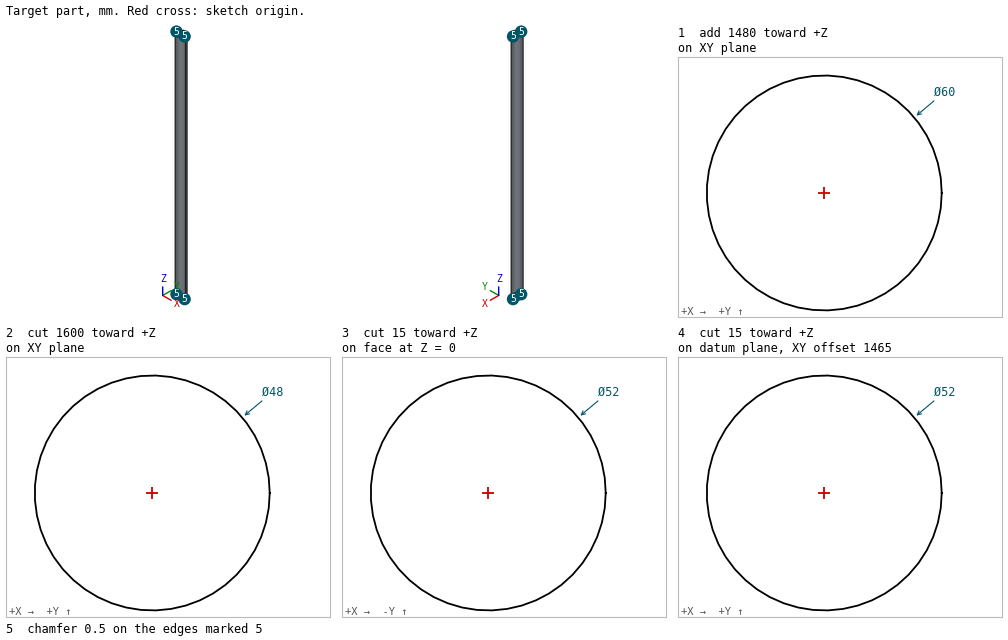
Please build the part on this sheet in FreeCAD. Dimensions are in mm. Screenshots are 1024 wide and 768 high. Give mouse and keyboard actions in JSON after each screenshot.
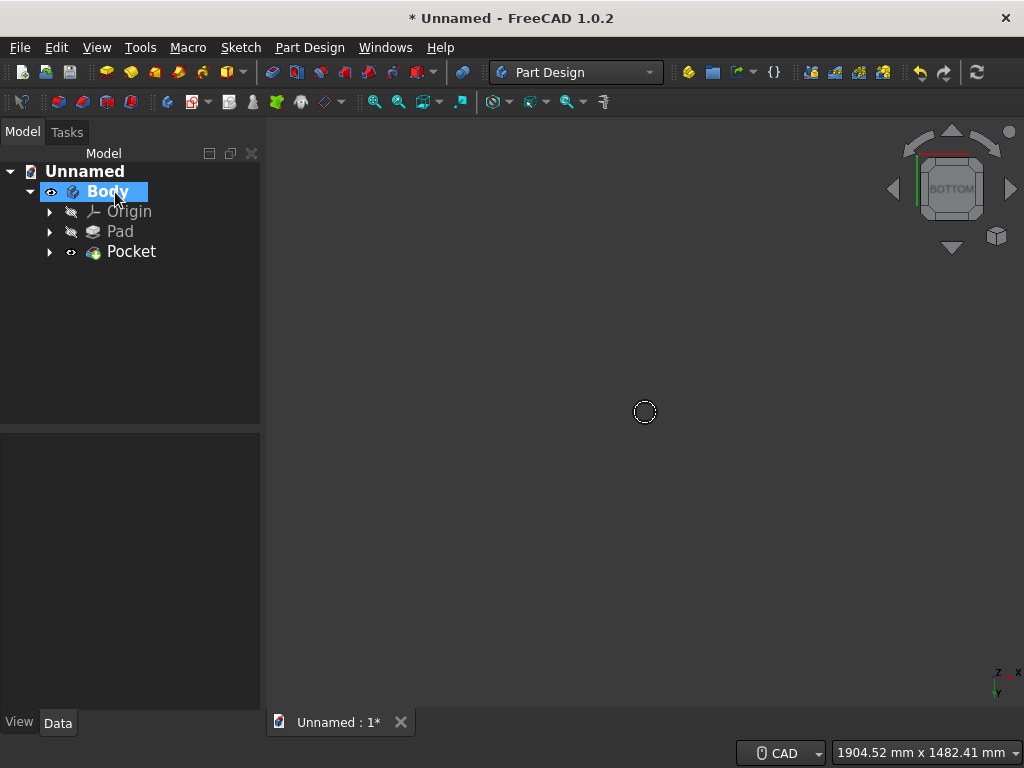
{"action": "left_click", "coordinate": [376, 102]}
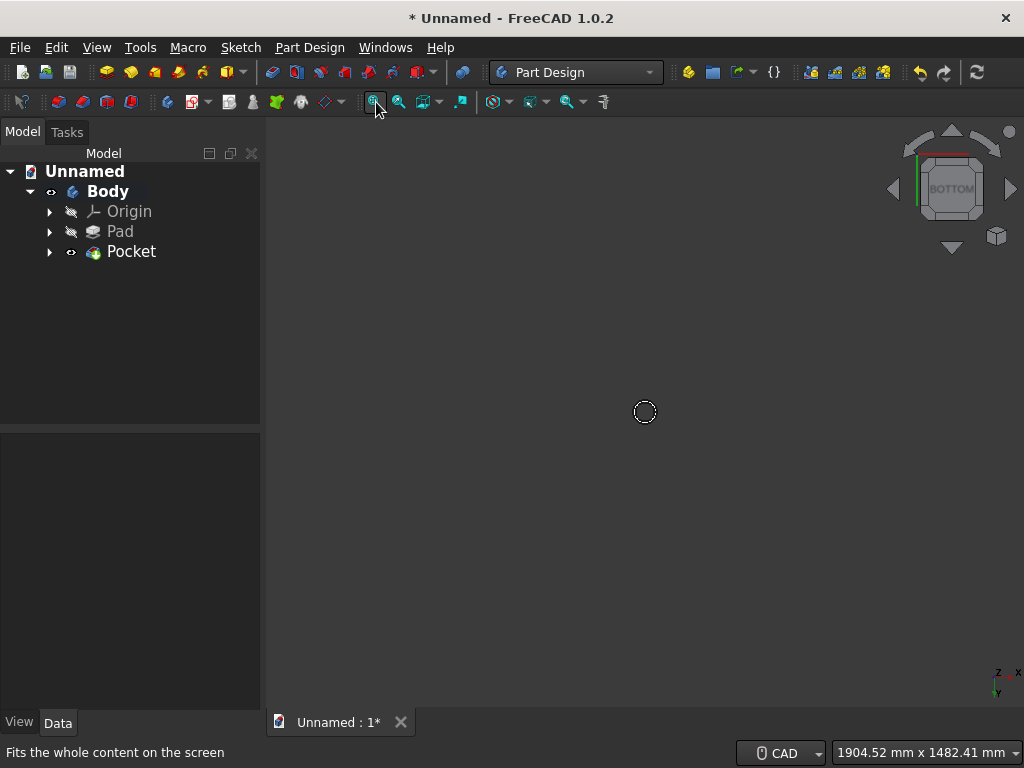
{"action": "scroll", "coordinate": [648, 421], "scroll_direction": "up", "scroll_amount": 12}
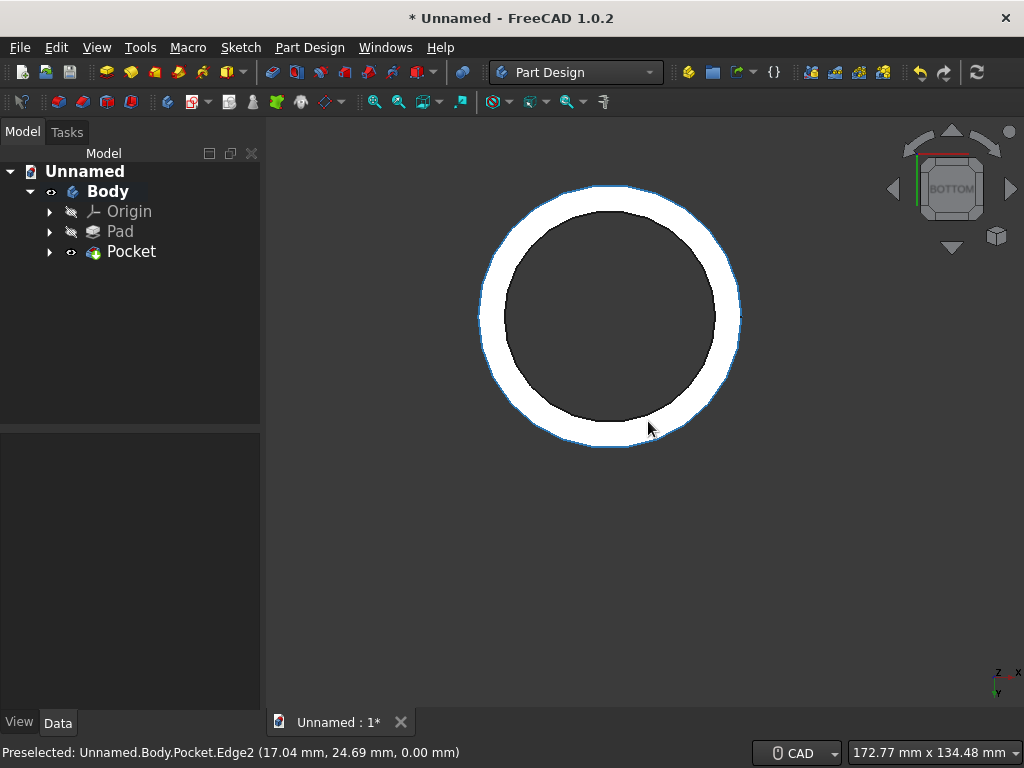
{"action": "left_click", "coordinate": [647, 428]}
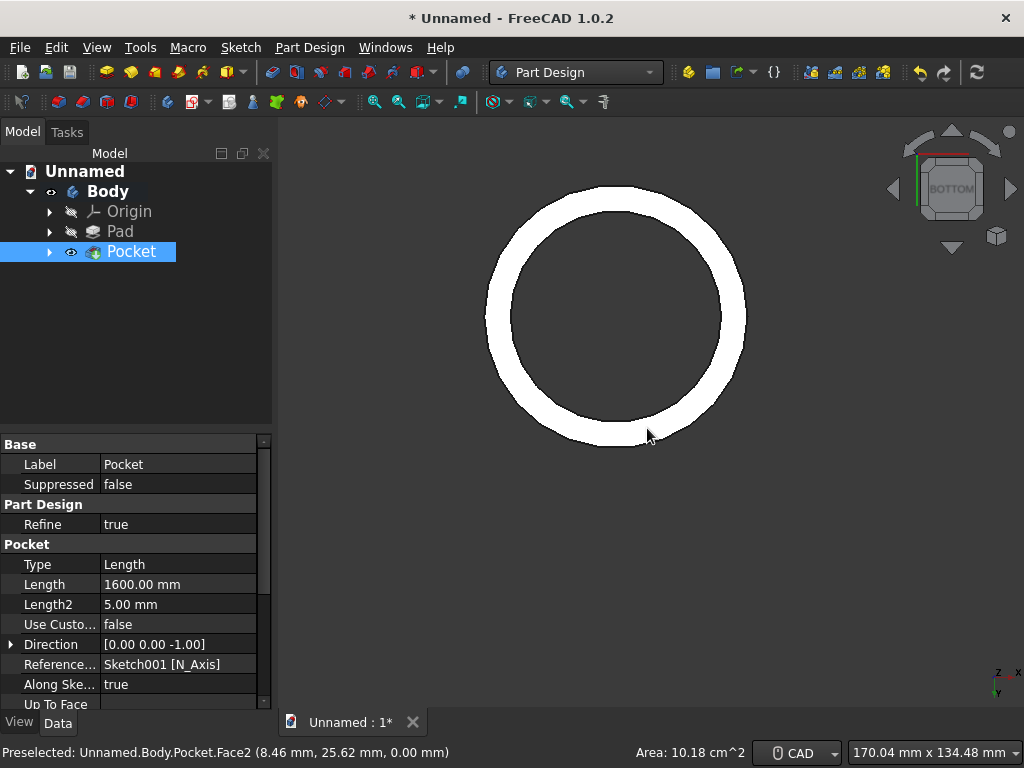
{"action": "left_click", "coordinate": [192, 102]}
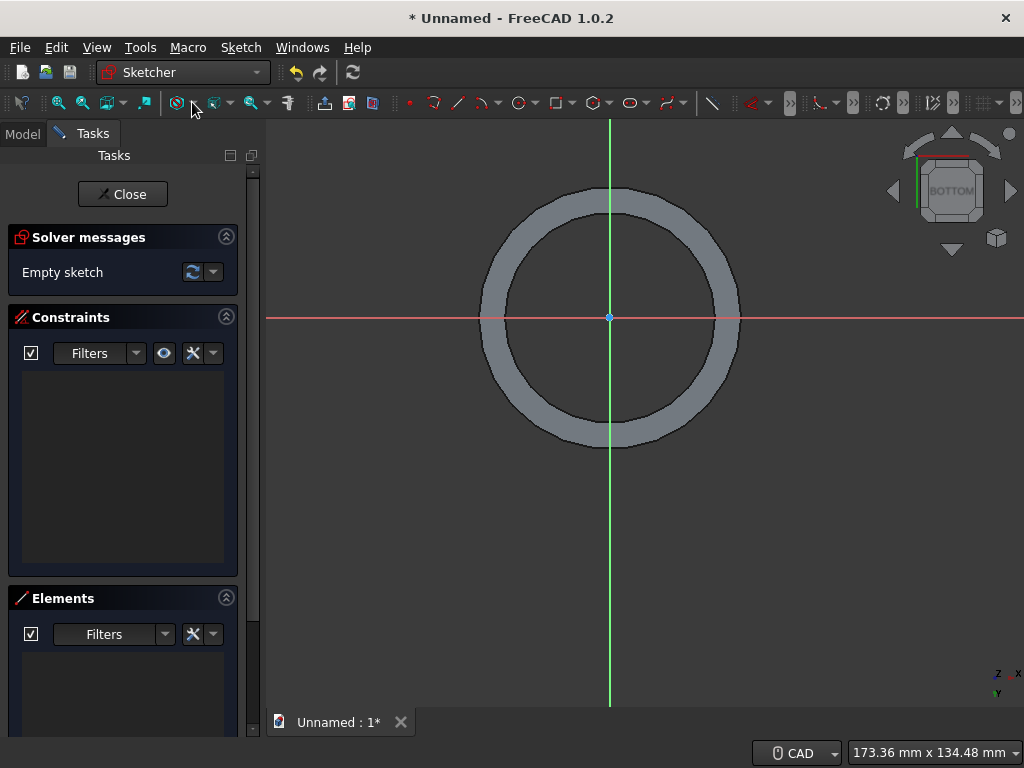
{"action": "scroll", "coordinate": [651, 202], "scroll_direction": "up", "scroll_amount": 3}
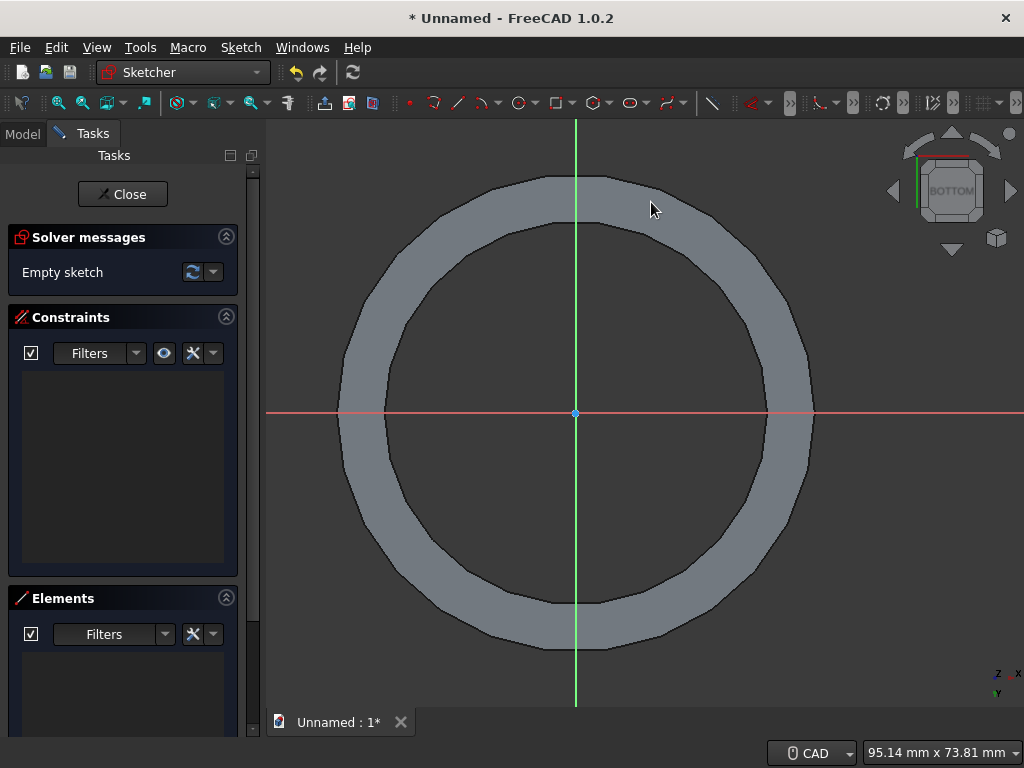
{"action": "left_click", "coordinate": [520, 104]}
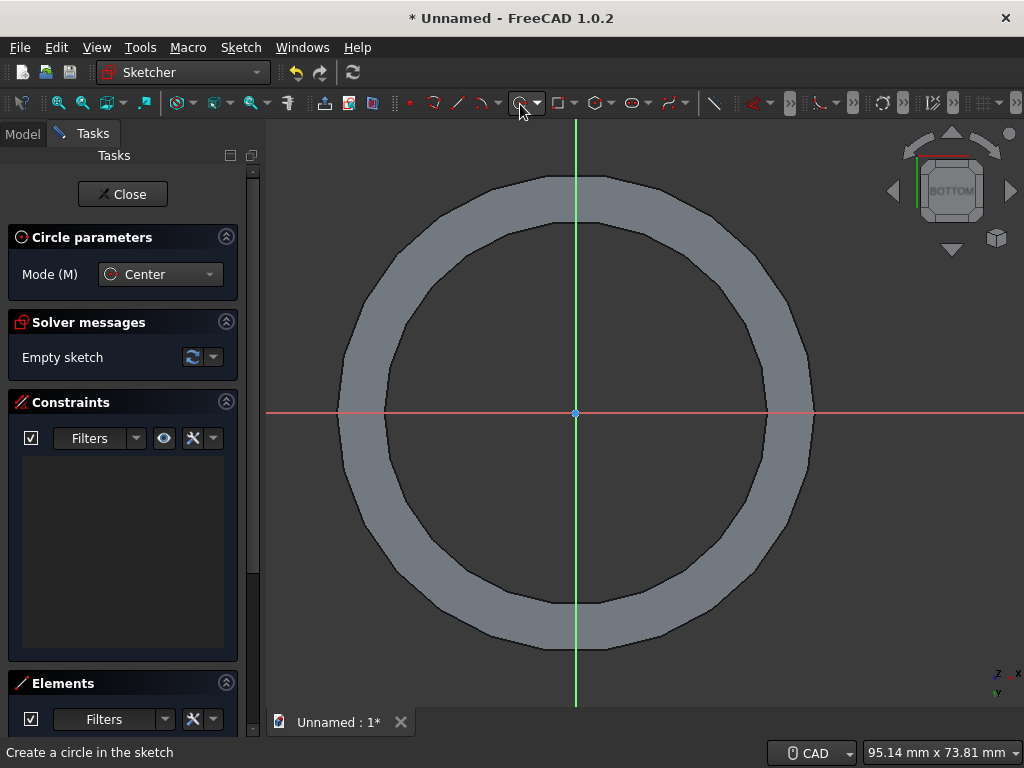
{"action": "left_click", "coordinate": [576, 413]}
{"action": "mouse_move", "coordinate": [722, 267]}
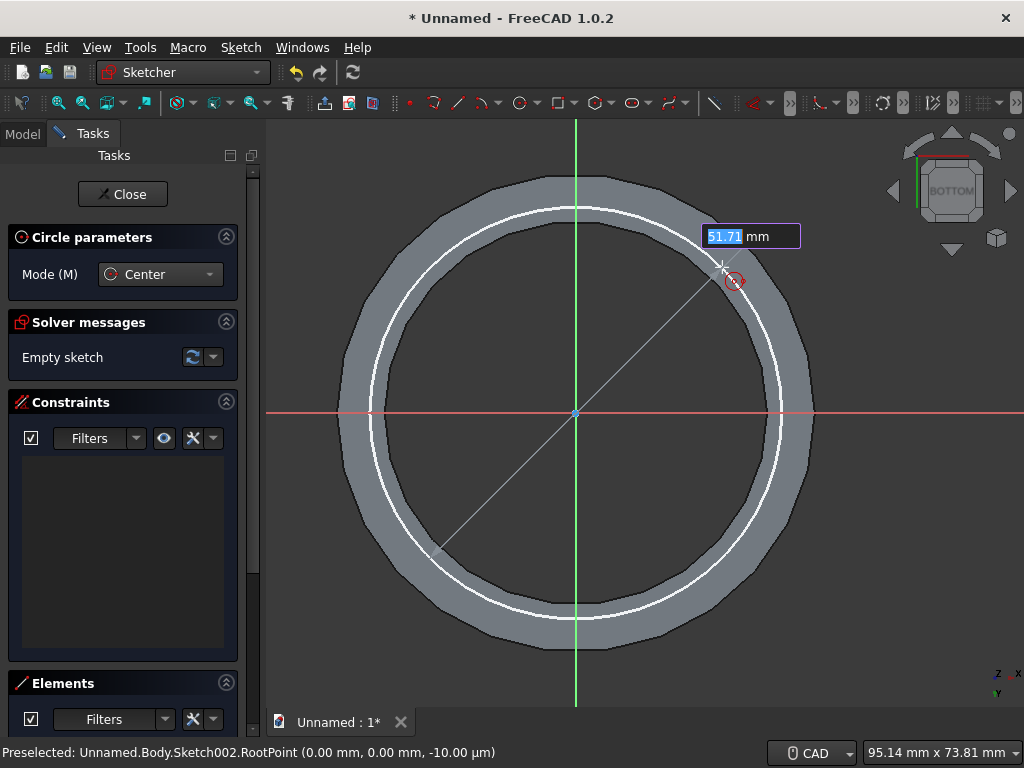
{"action": "type", "text": "52"}
{"action": "key", "text": "Return"}
{"action": "key", "text": "Escape"}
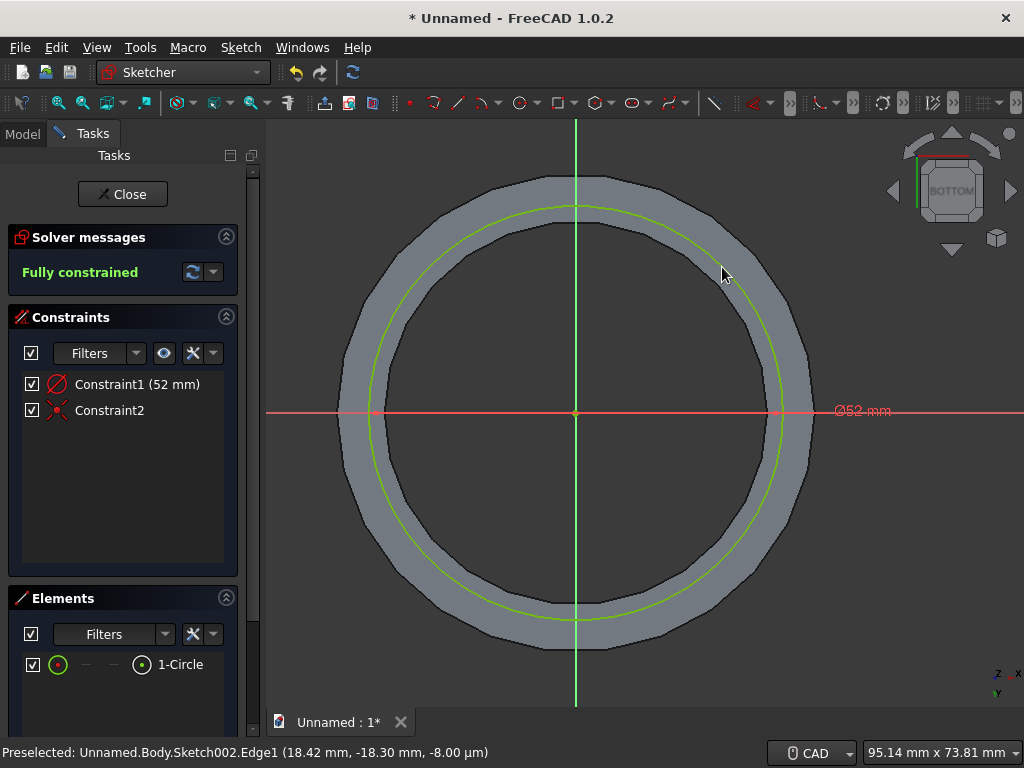
{"action": "left_click", "coordinate": [123, 194]}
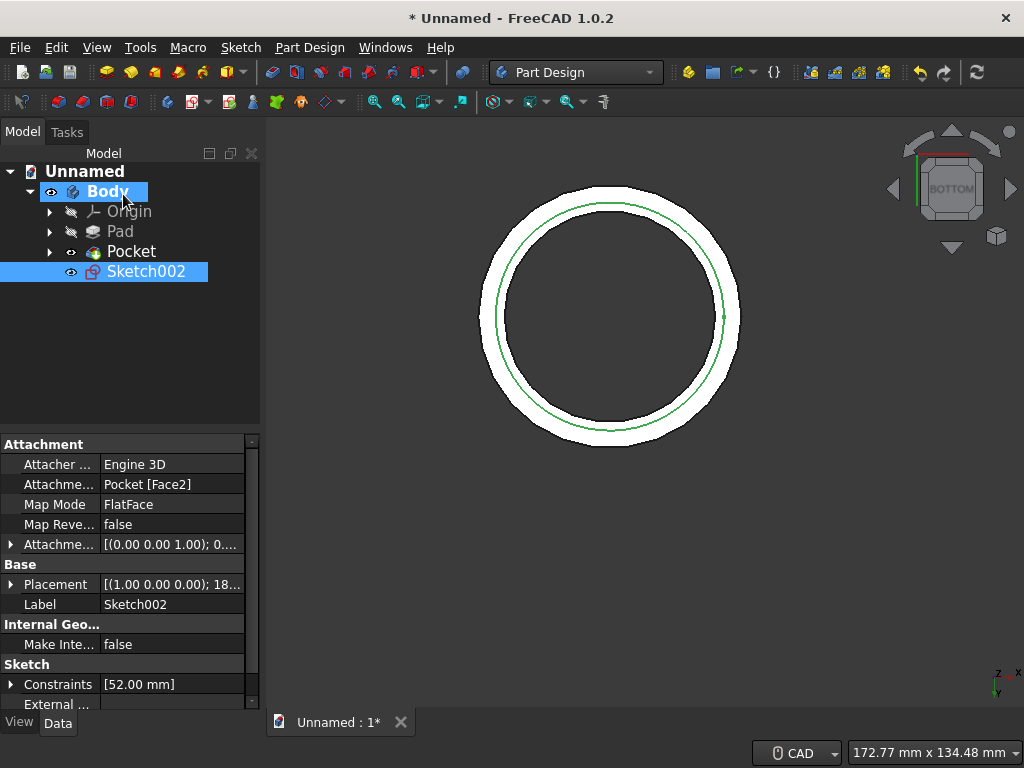
{"action": "left_click", "coordinate": [274, 72]}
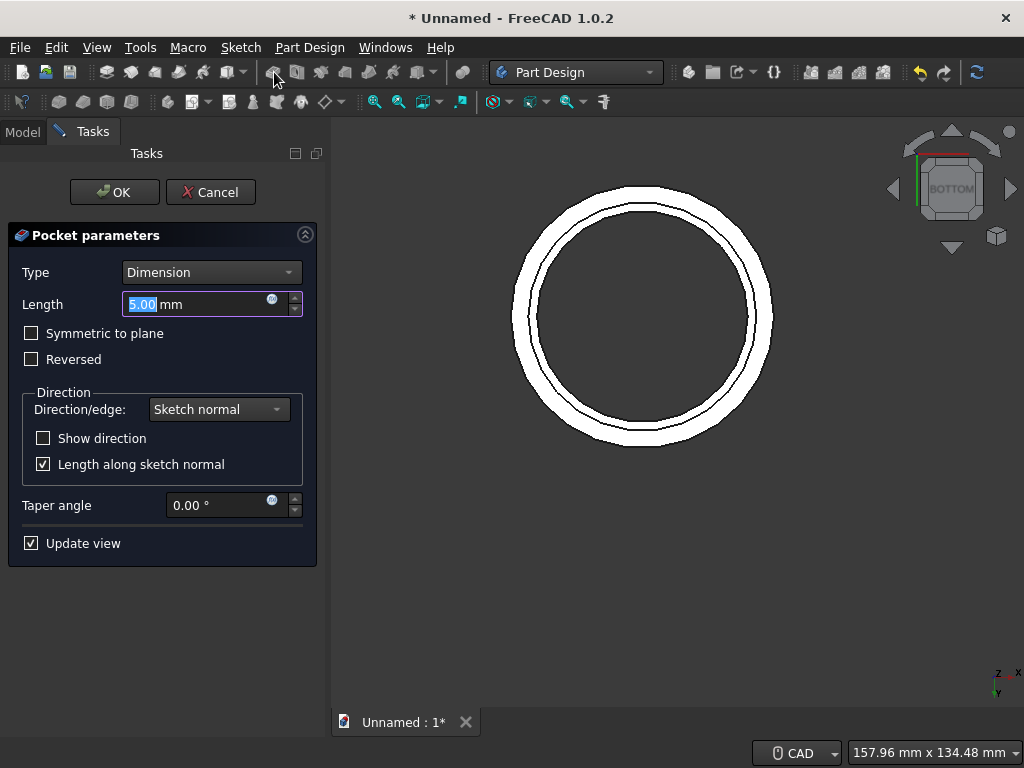
{"action": "type", "text": "15"}
{"action": "key", "text": "Tab"}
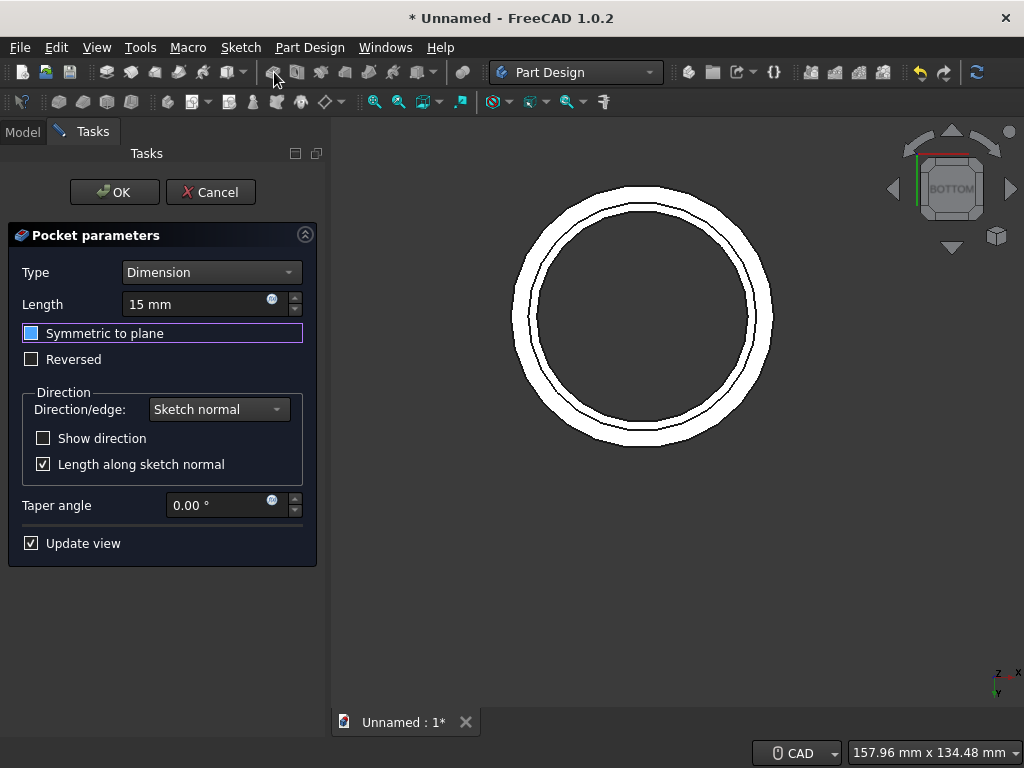
{"action": "left_click", "coordinate": [115, 192]}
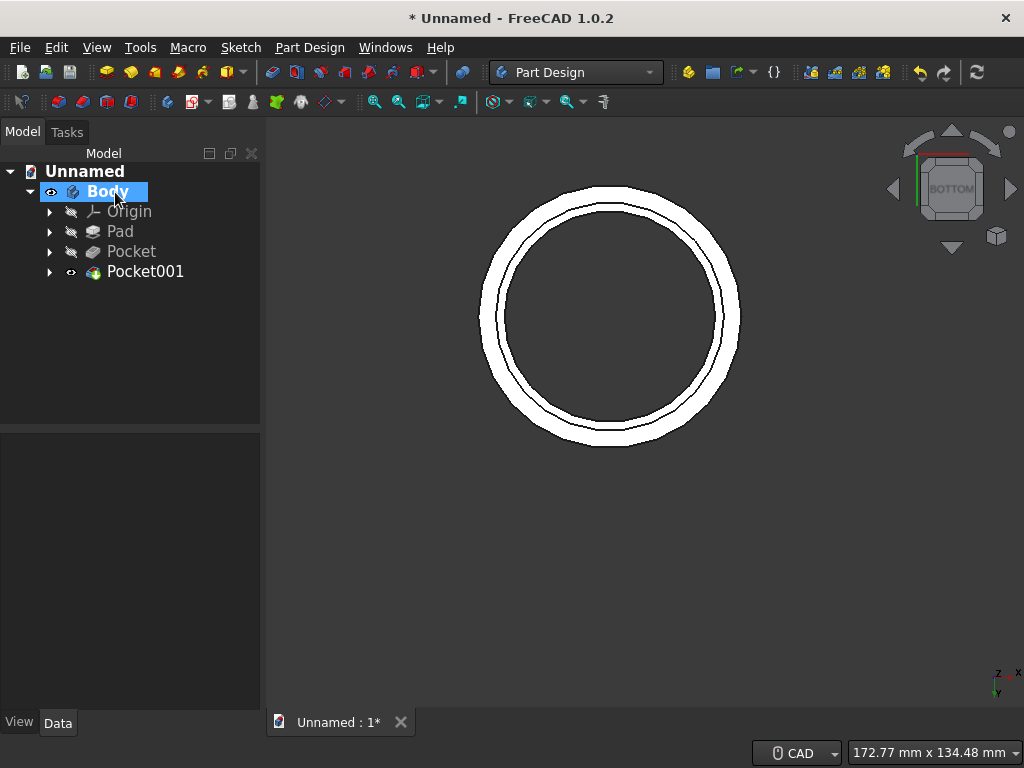
{"action": "left_click", "coordinate": [376, 102]}